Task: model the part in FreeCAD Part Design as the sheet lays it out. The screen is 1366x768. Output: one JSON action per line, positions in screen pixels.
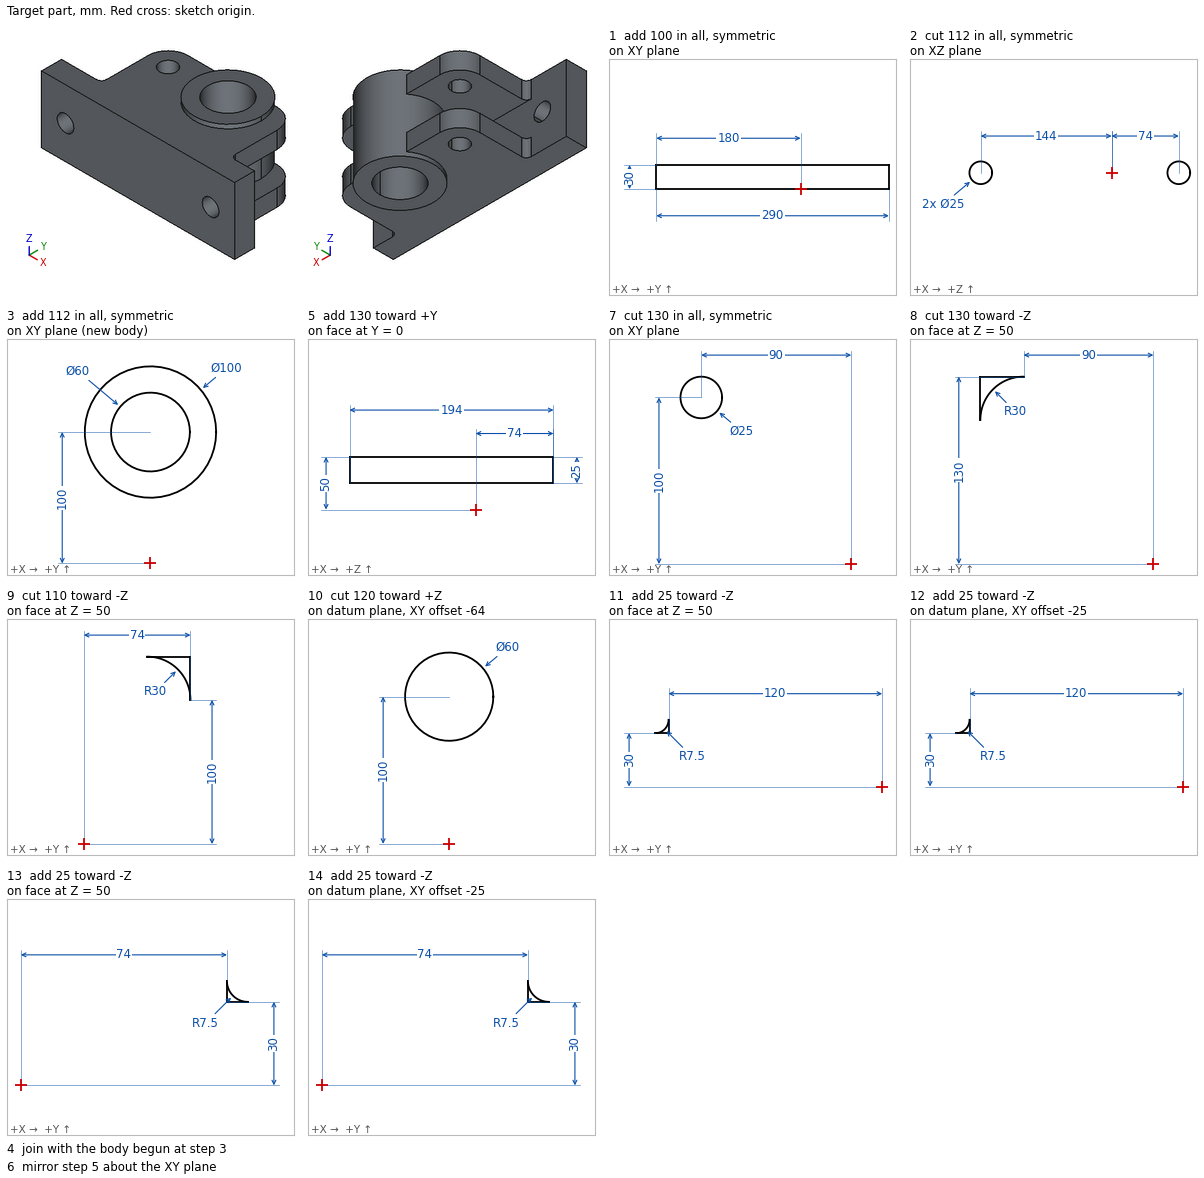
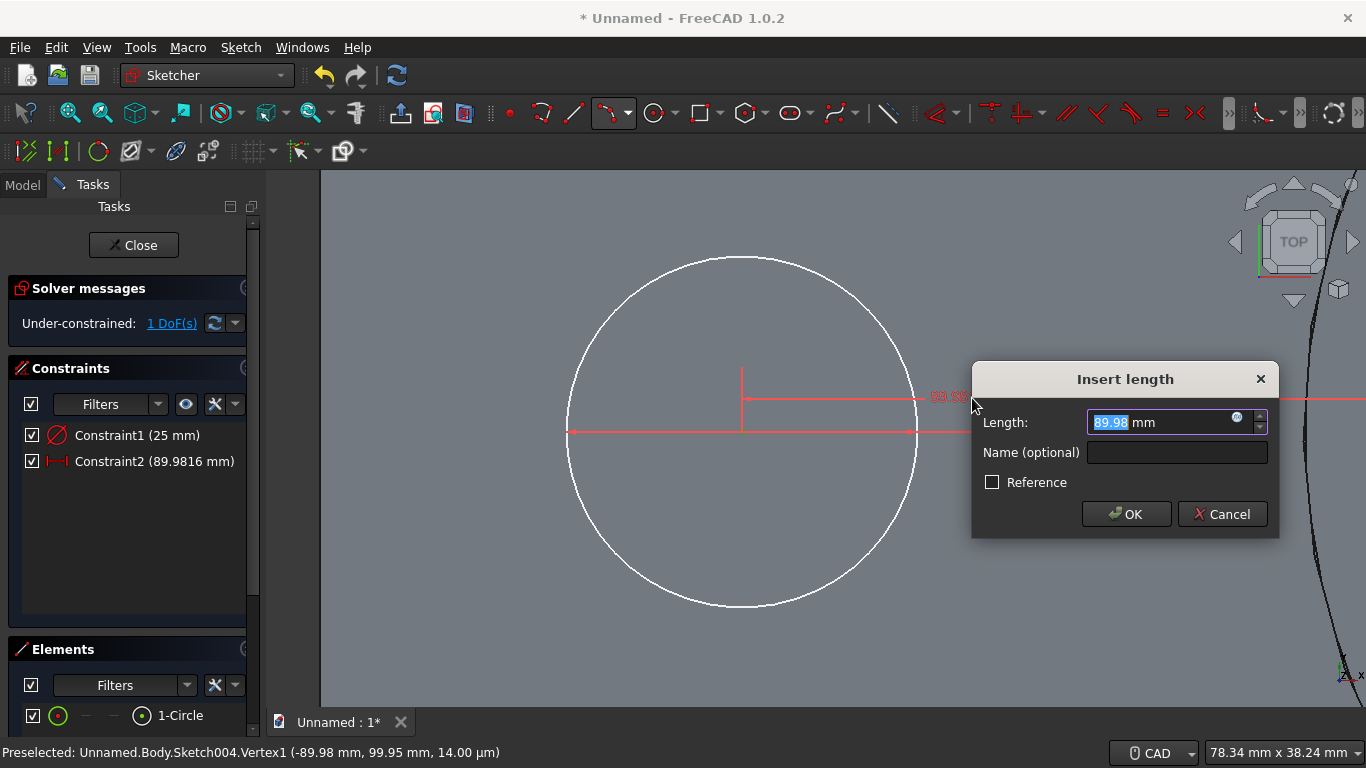
{"action": "type", "text": "90"}
{"action": "key", "text": "Return"}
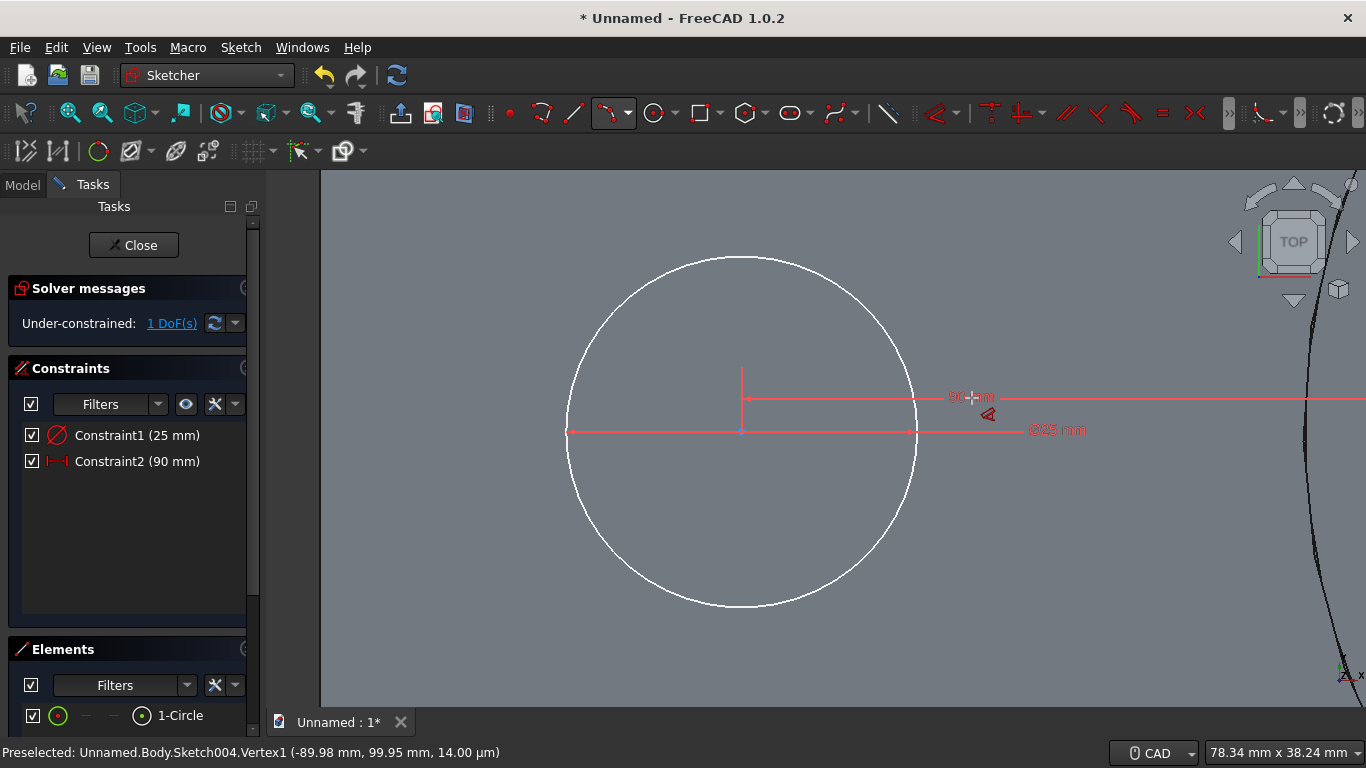
{"action": "left_click", "coordinate": [742, 432]}
{"action": "left_click", "coordinate": [708, 556]}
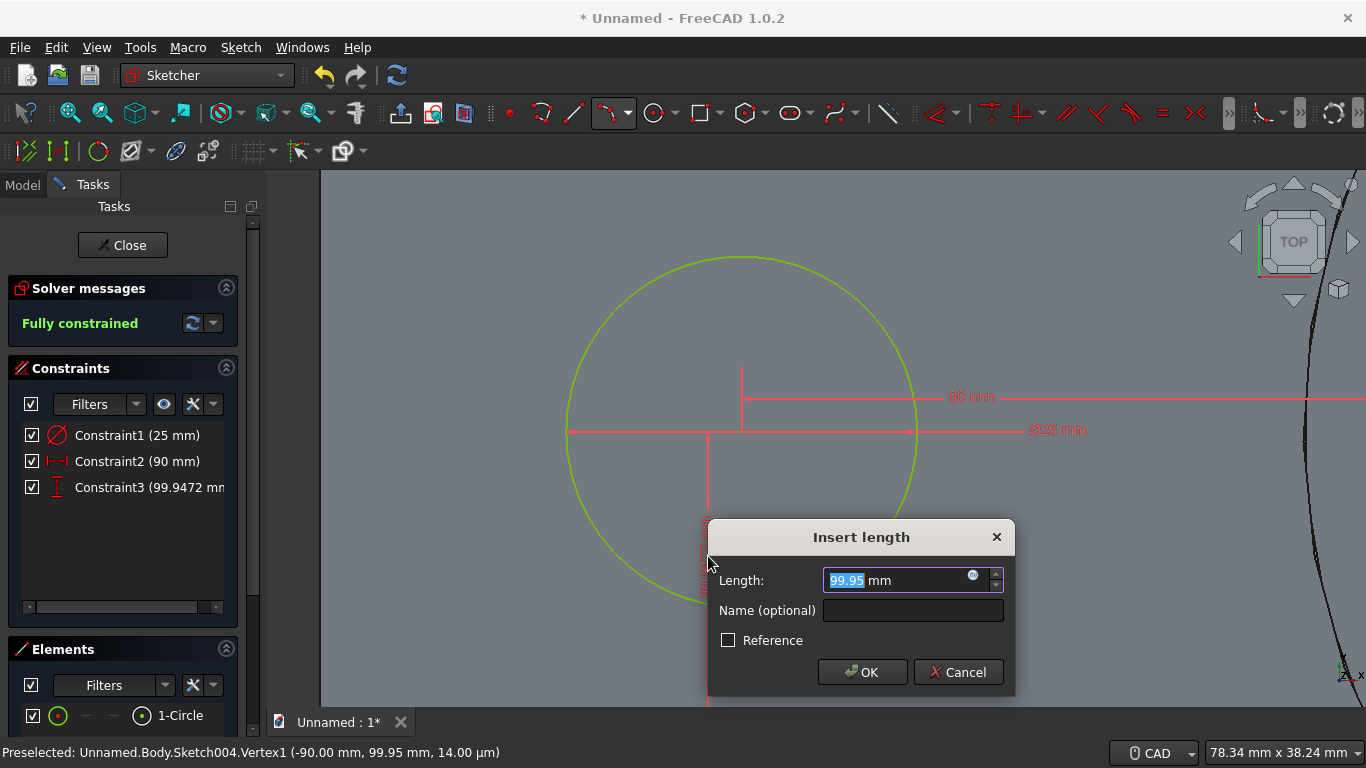
{"action": "type", "text": "100"}
{"action": "key", "text": "Return"}
{"action": "key", "text": "Escape"}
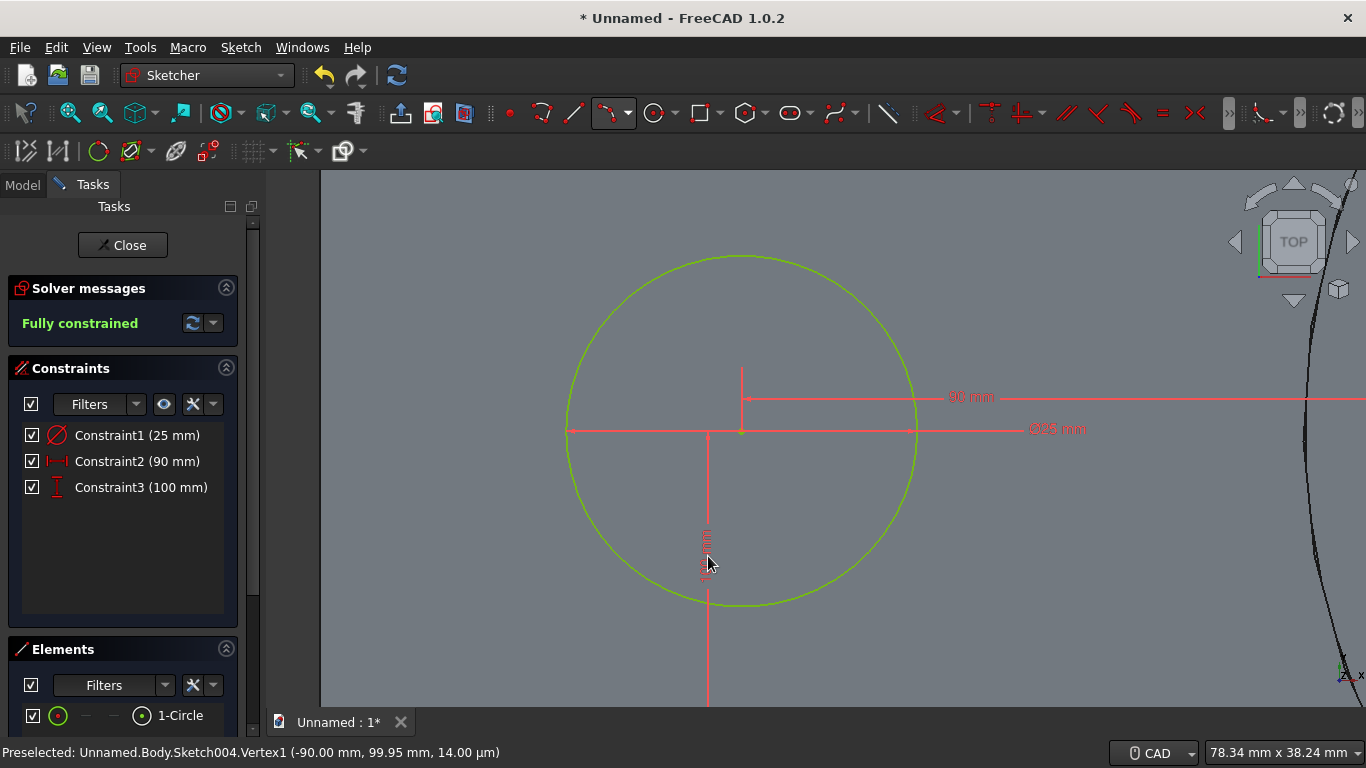
{"action": "left_click", "coordinate": [123, 245]}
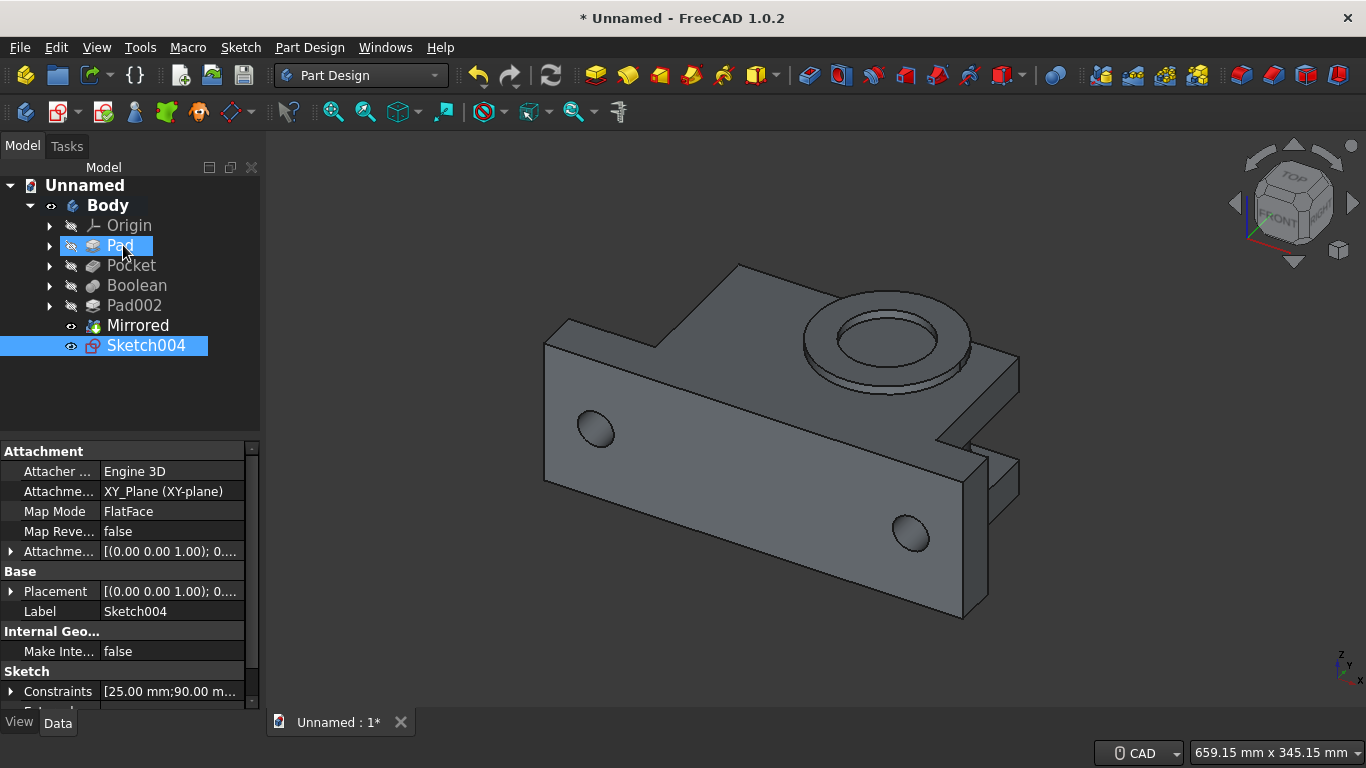
{"action": "left_click", "coordinate": [810, 76]}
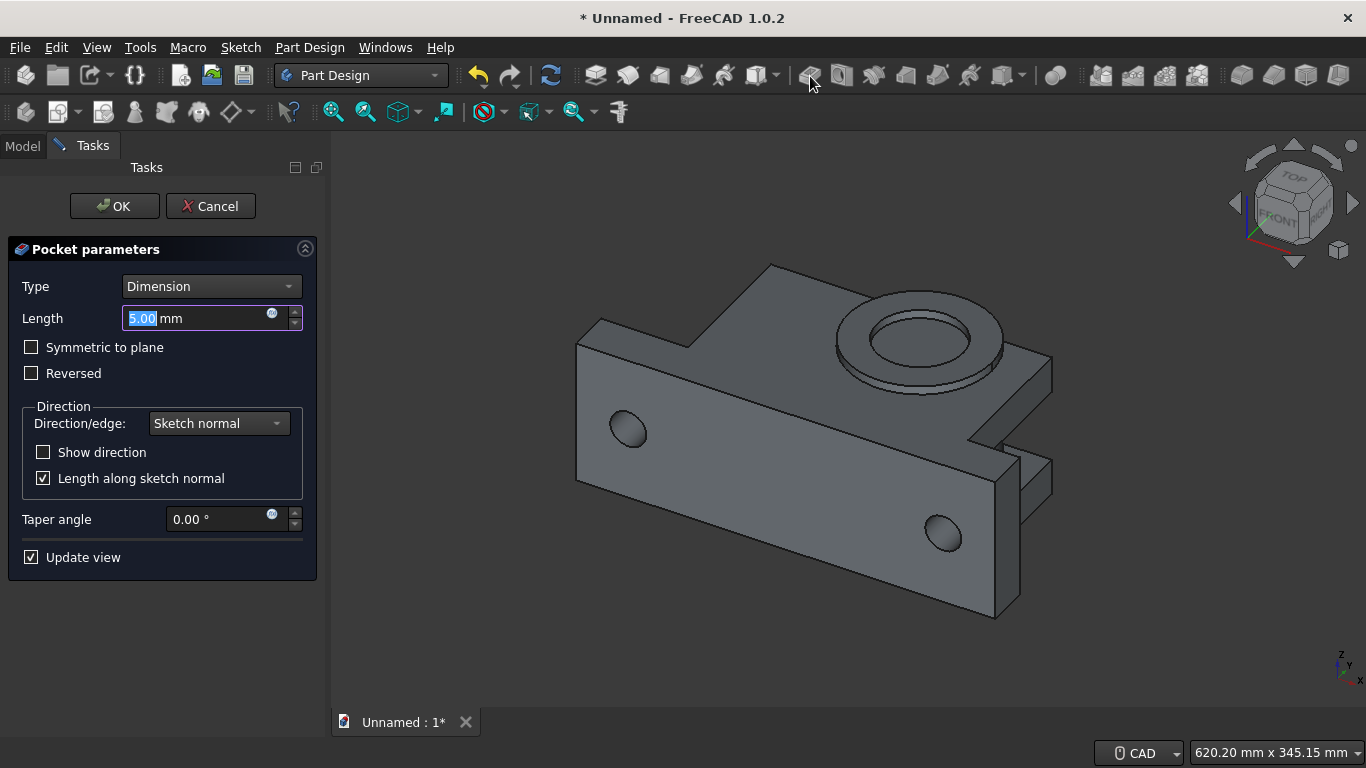
{"action": "type", "text": "130"}
{"action": "key", "text": "Tab"}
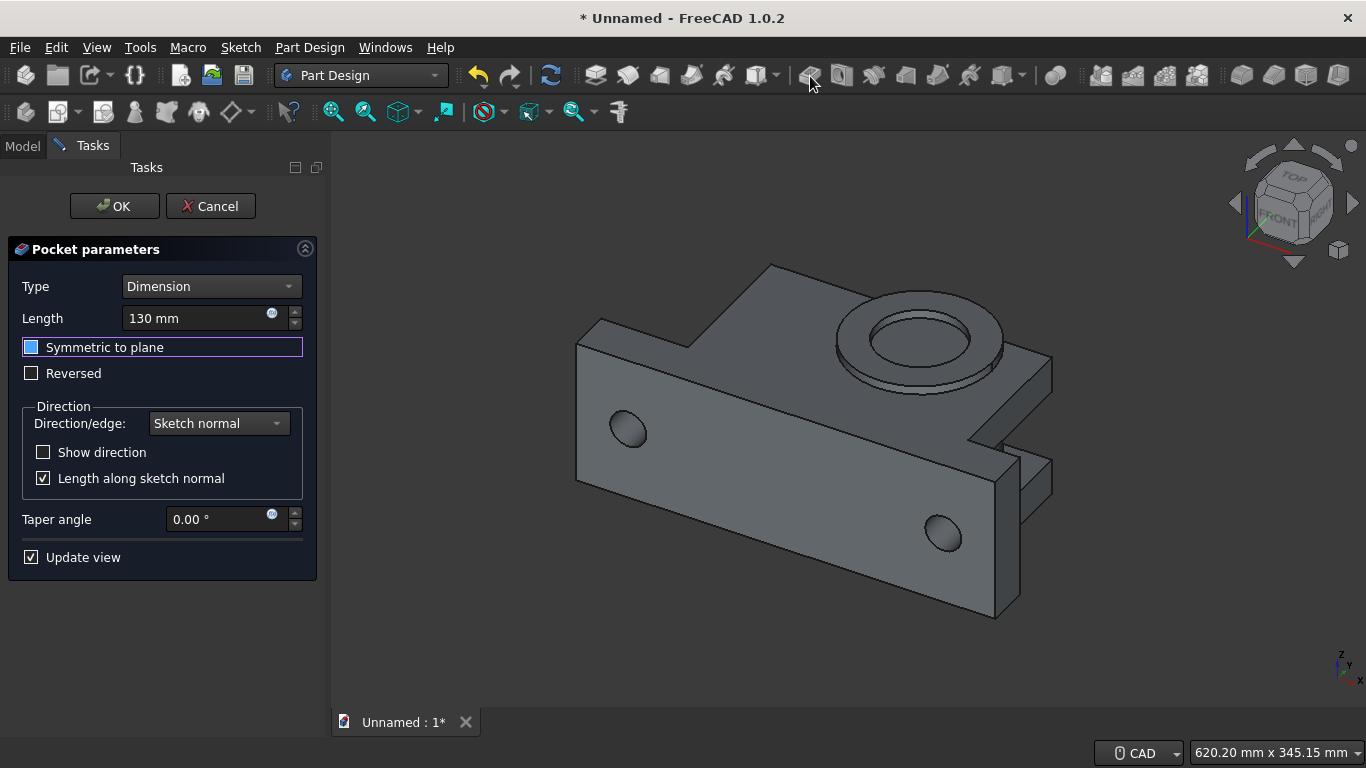
{"action": "left_click", "coordinate": [30, 347]}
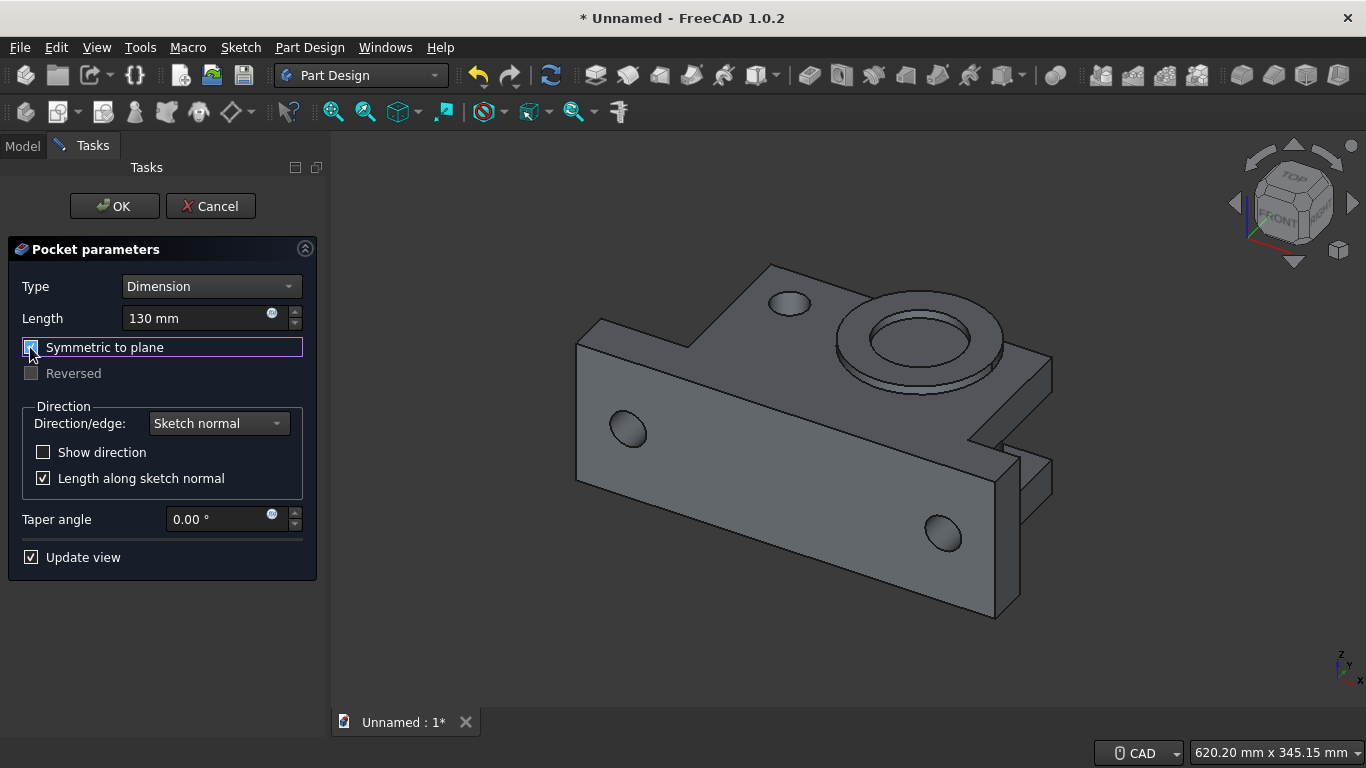
{"action": "left_click", "coordinate": [115, 206]}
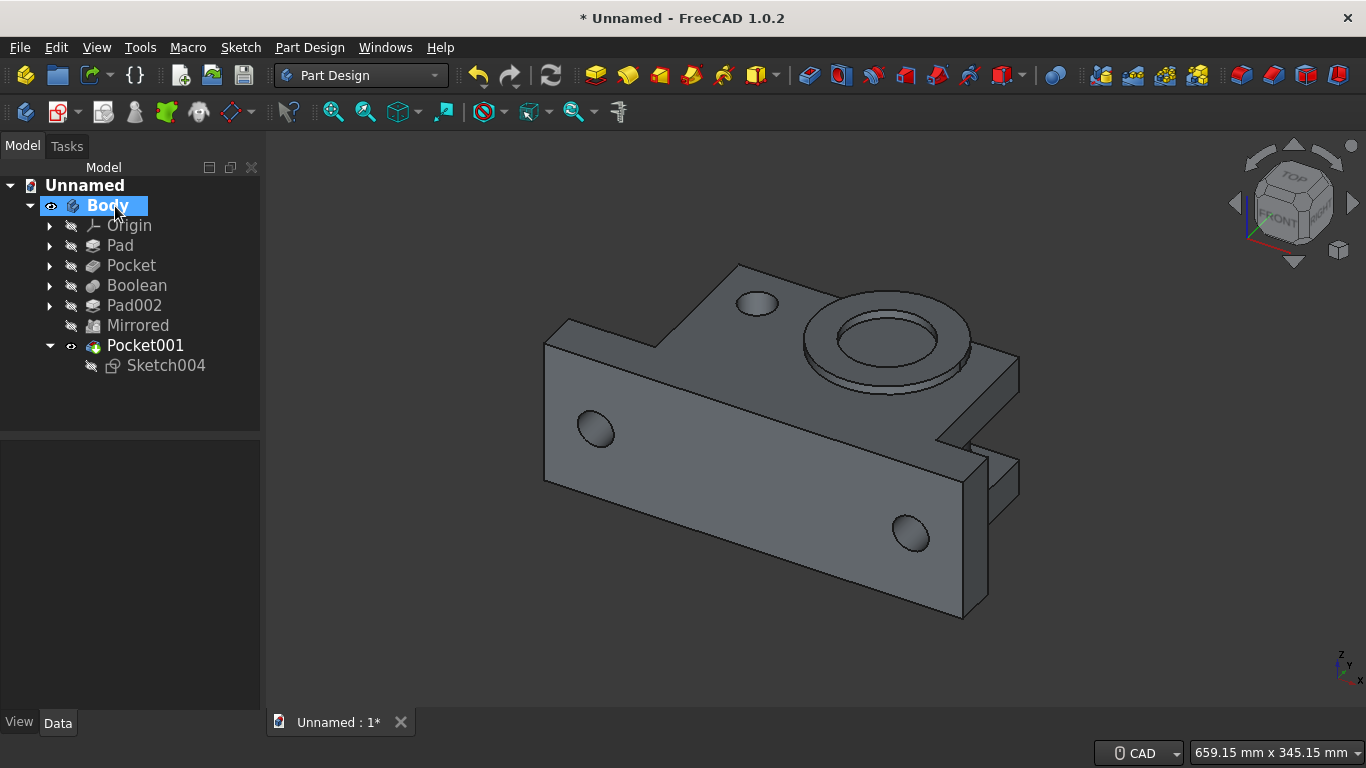
{"action": "left_click", "coordinate": [732, 354]}